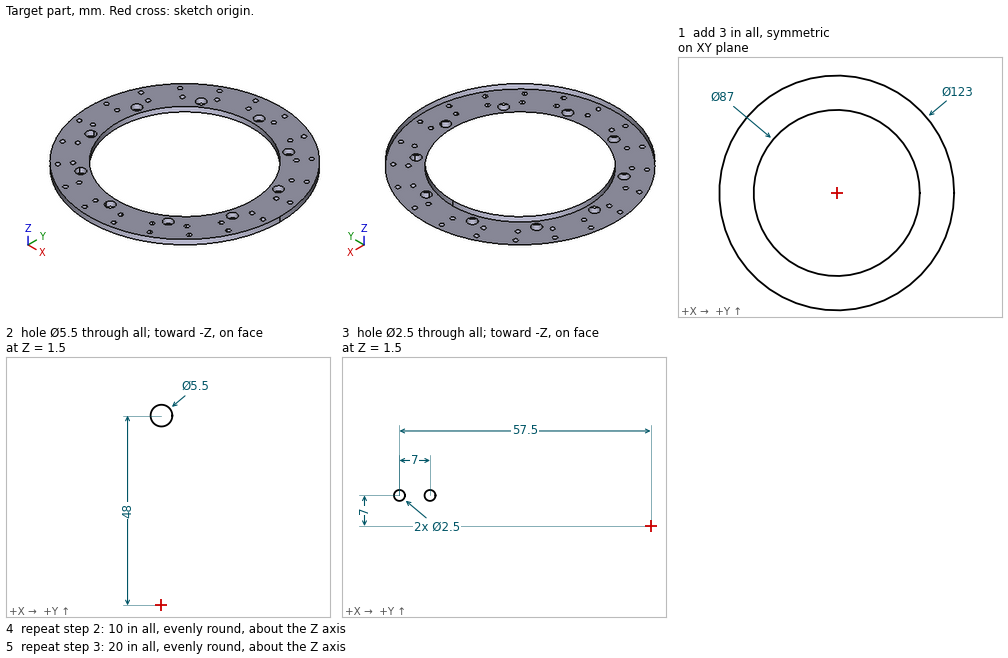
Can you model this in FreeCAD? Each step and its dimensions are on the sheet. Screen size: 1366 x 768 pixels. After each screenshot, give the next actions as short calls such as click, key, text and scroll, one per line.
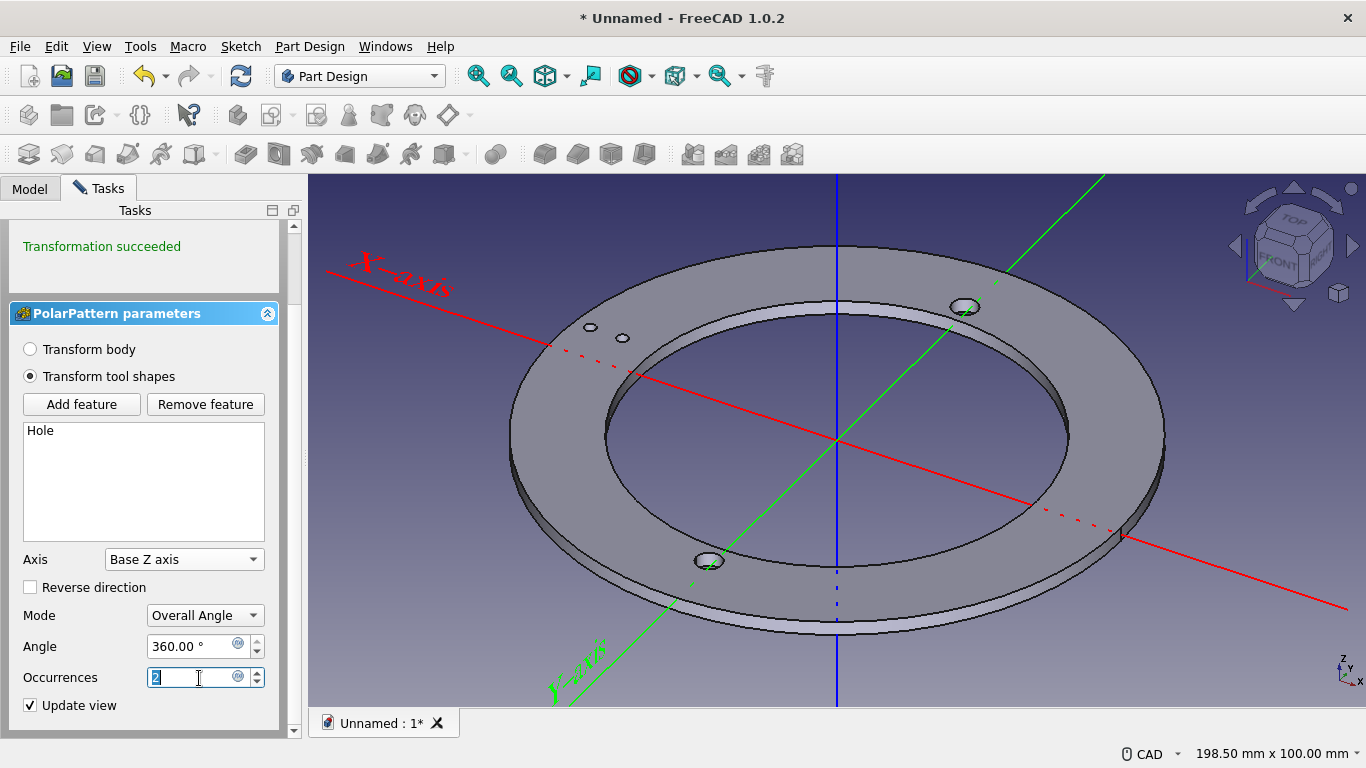
text(10)
key(Tab)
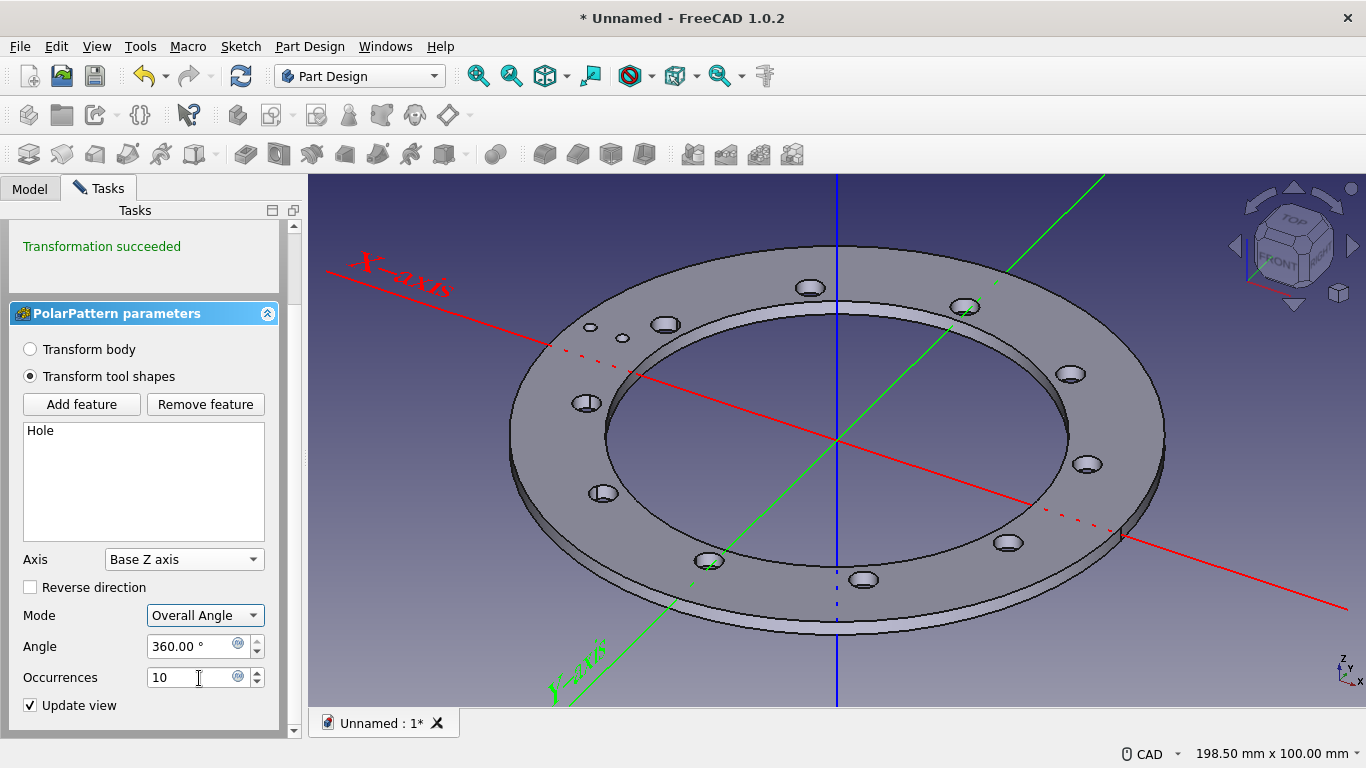
scroll(294, 479, up, 3)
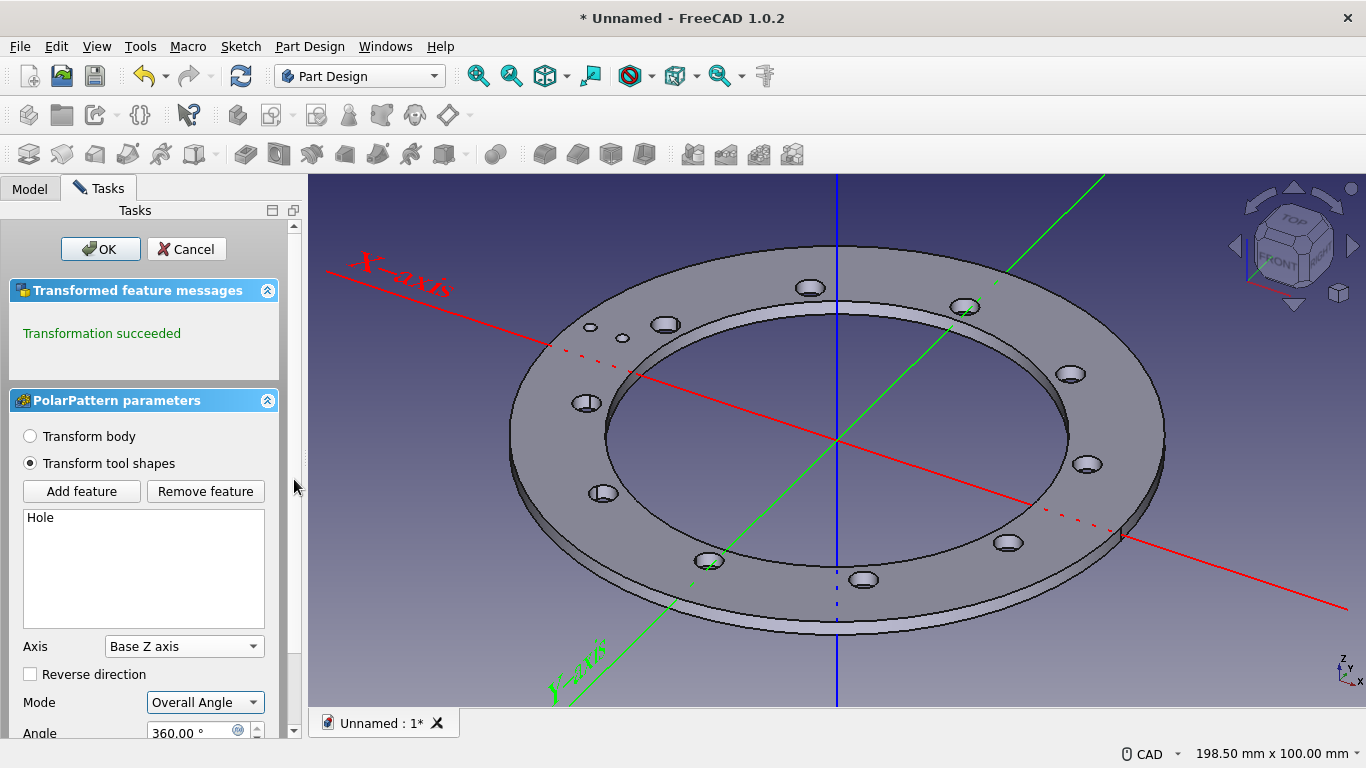
click(101, 249)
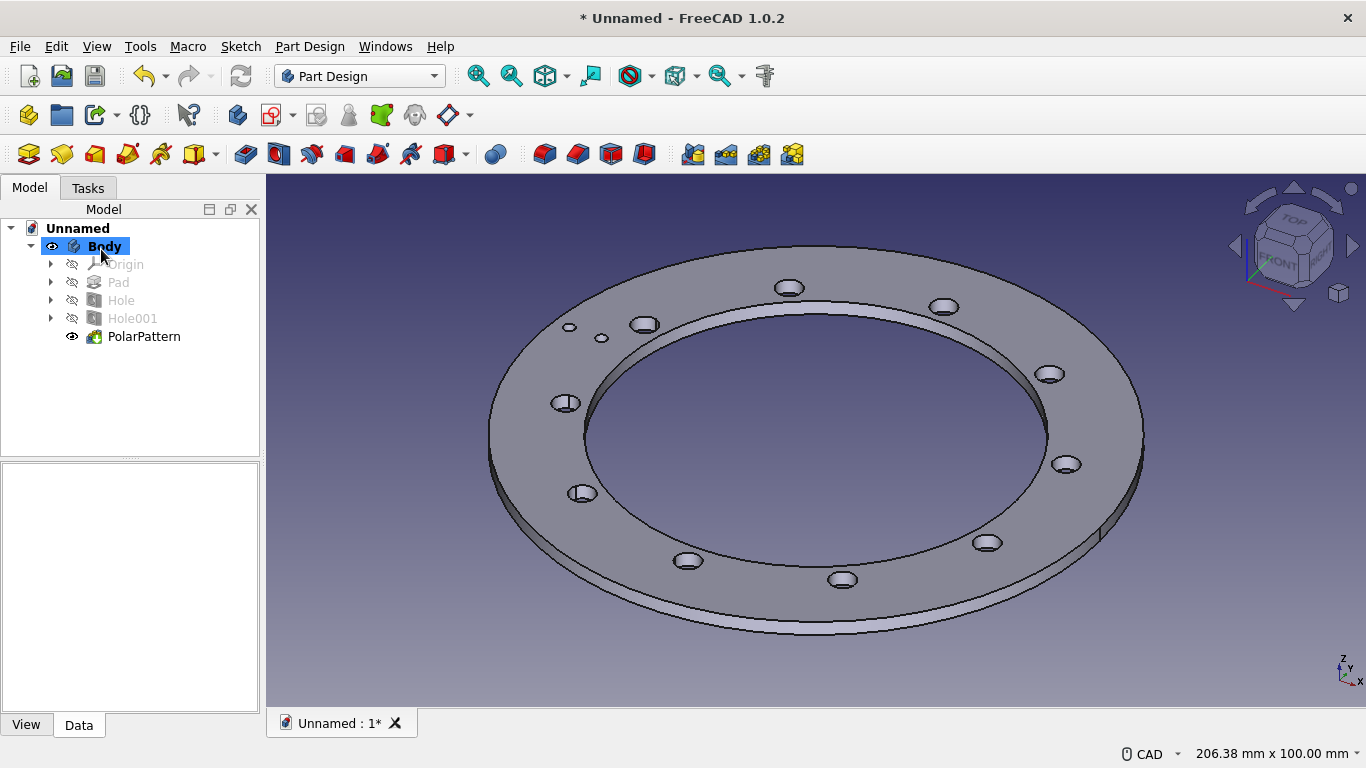
click(117, 318)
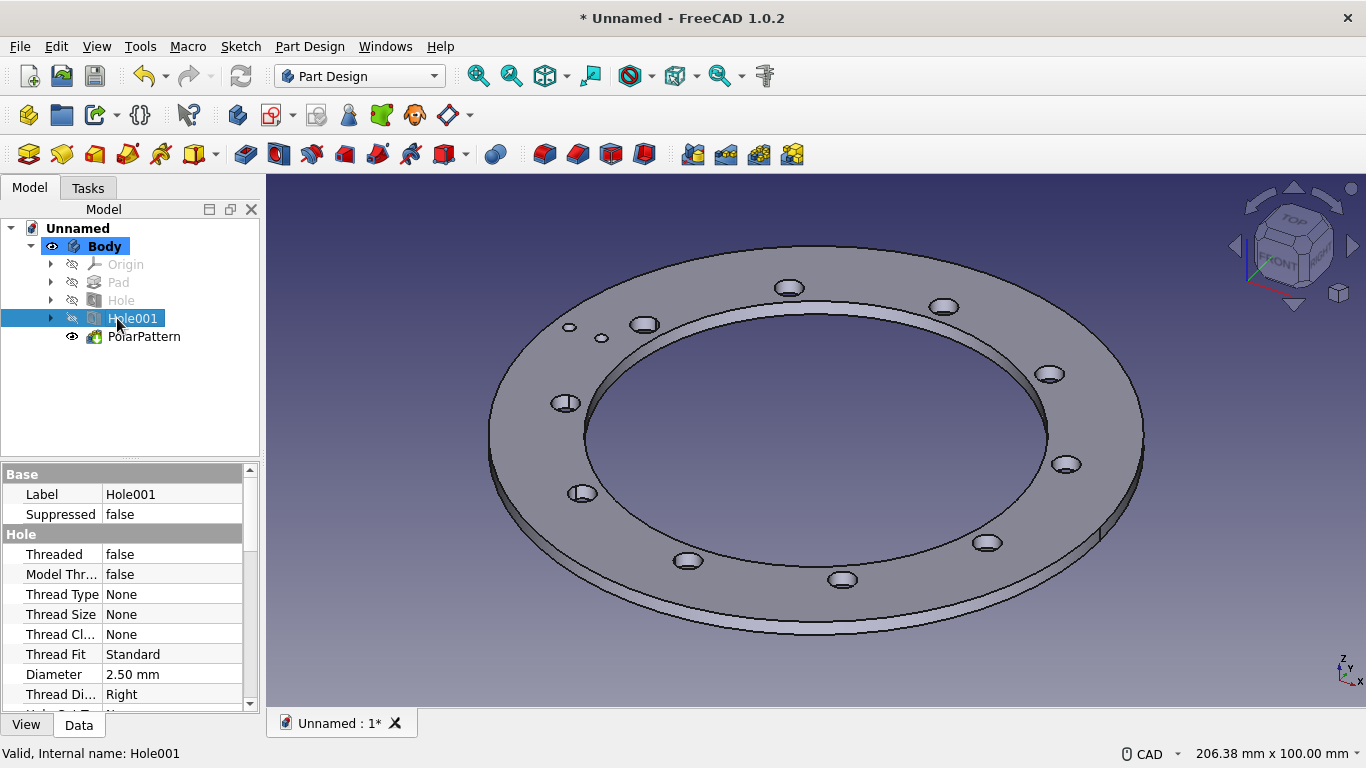
click(759, 154)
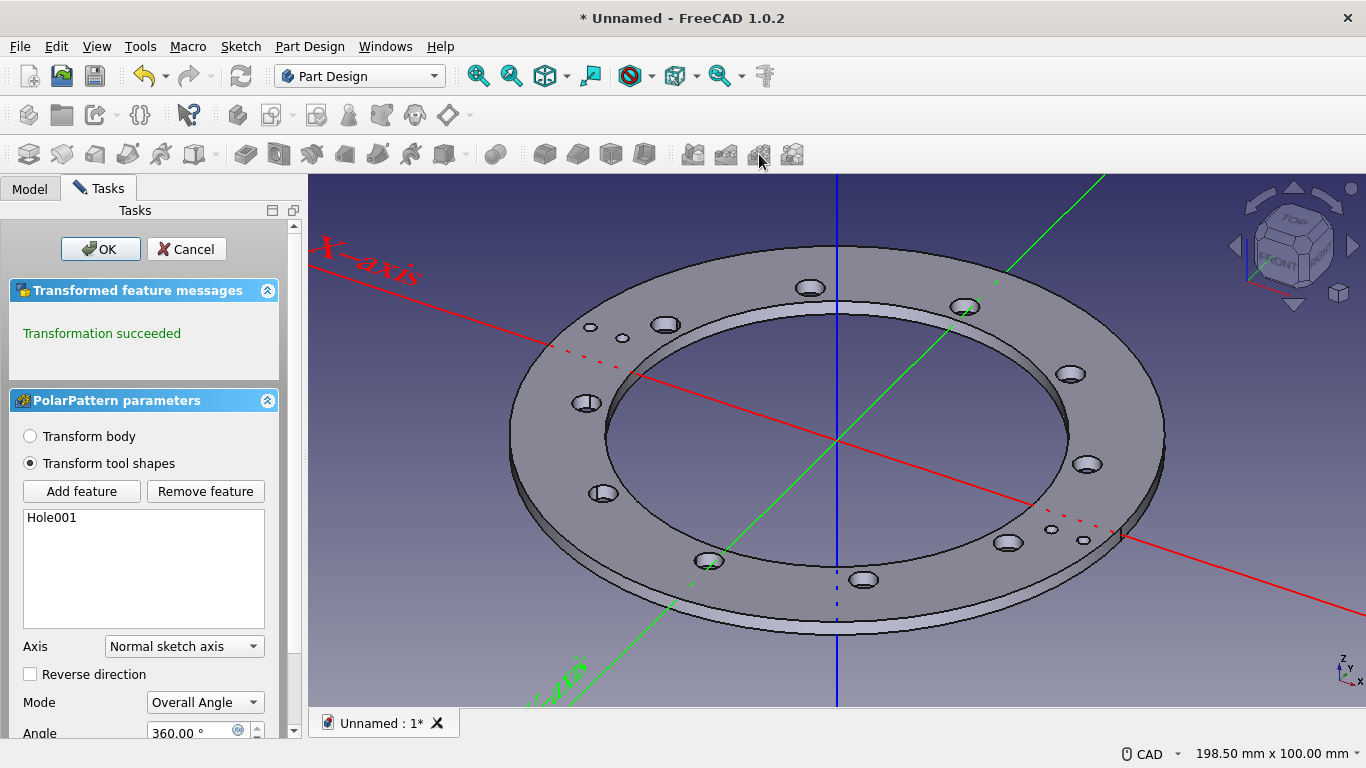
click(185, 646)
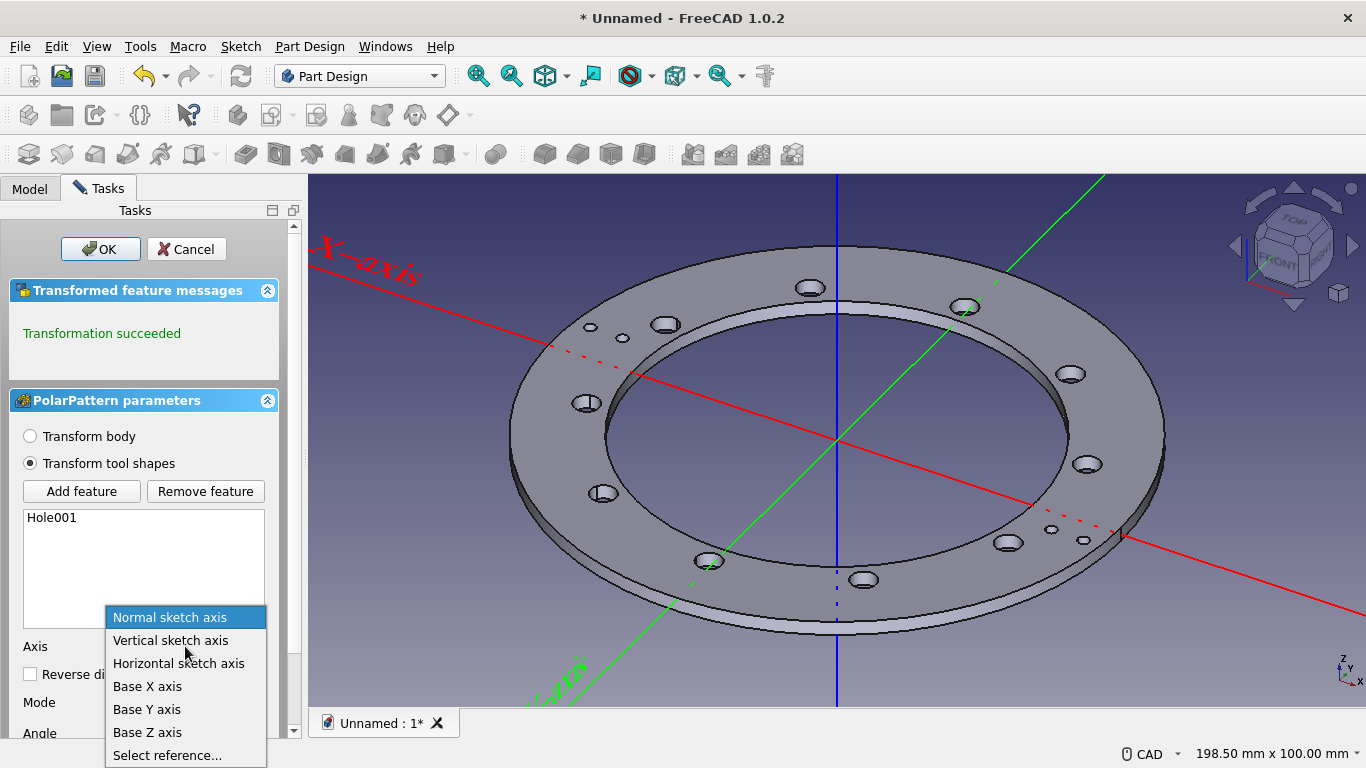
click(184, 732)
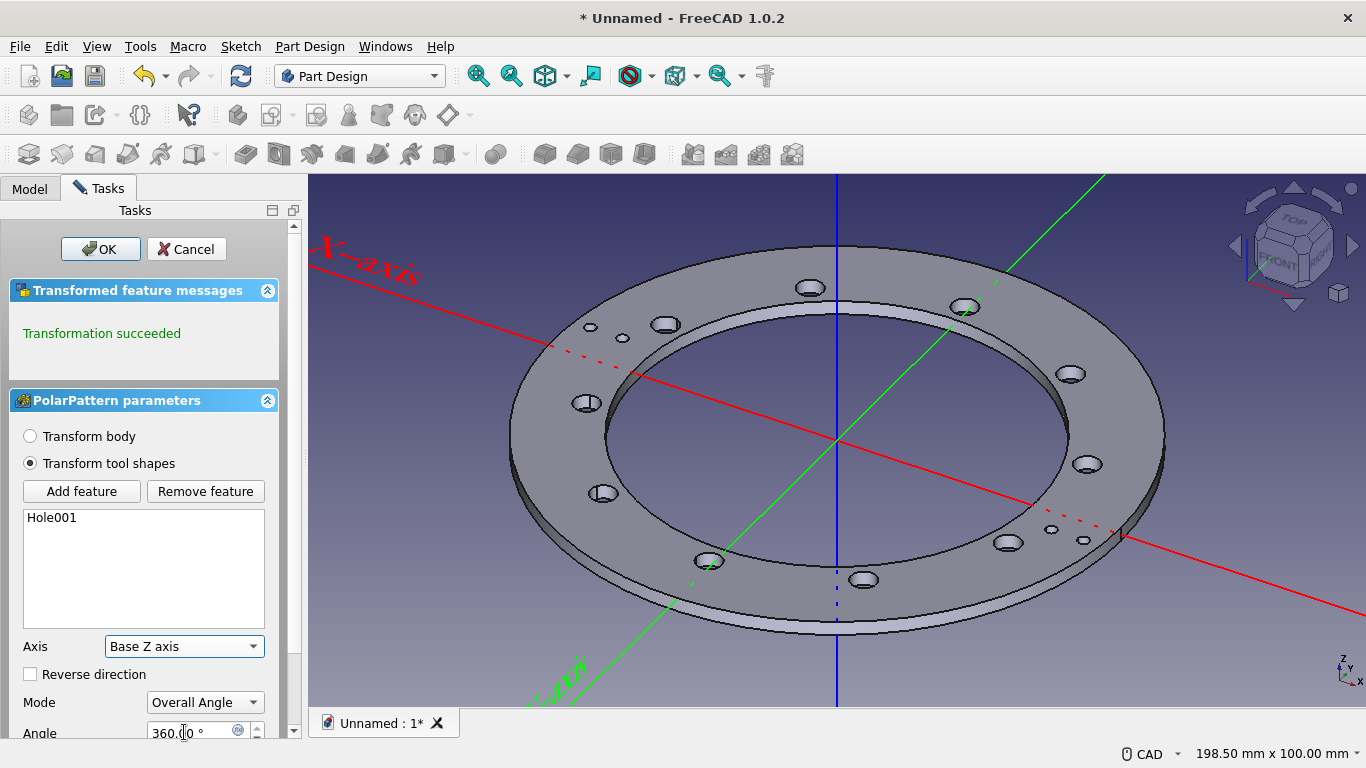
scroll(294, 479, down, 2)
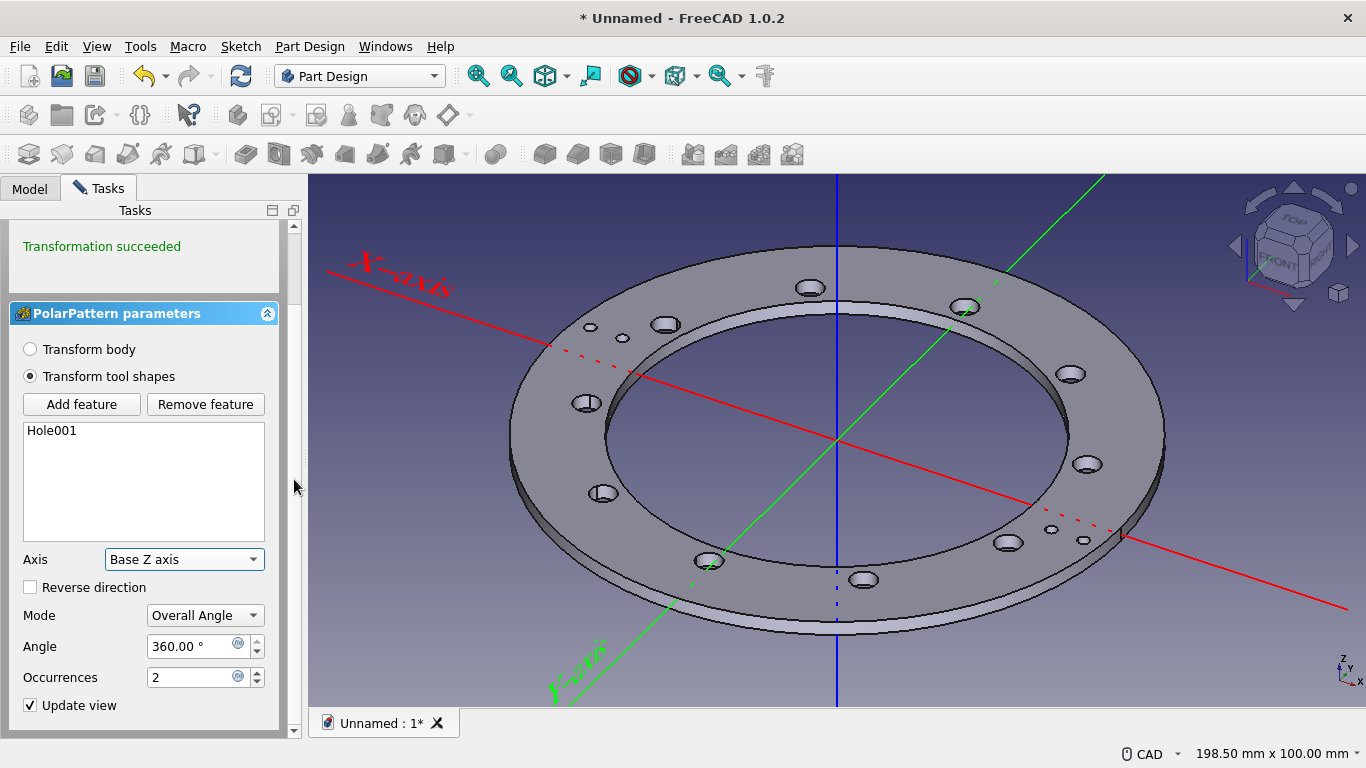
triple_click(199, 678)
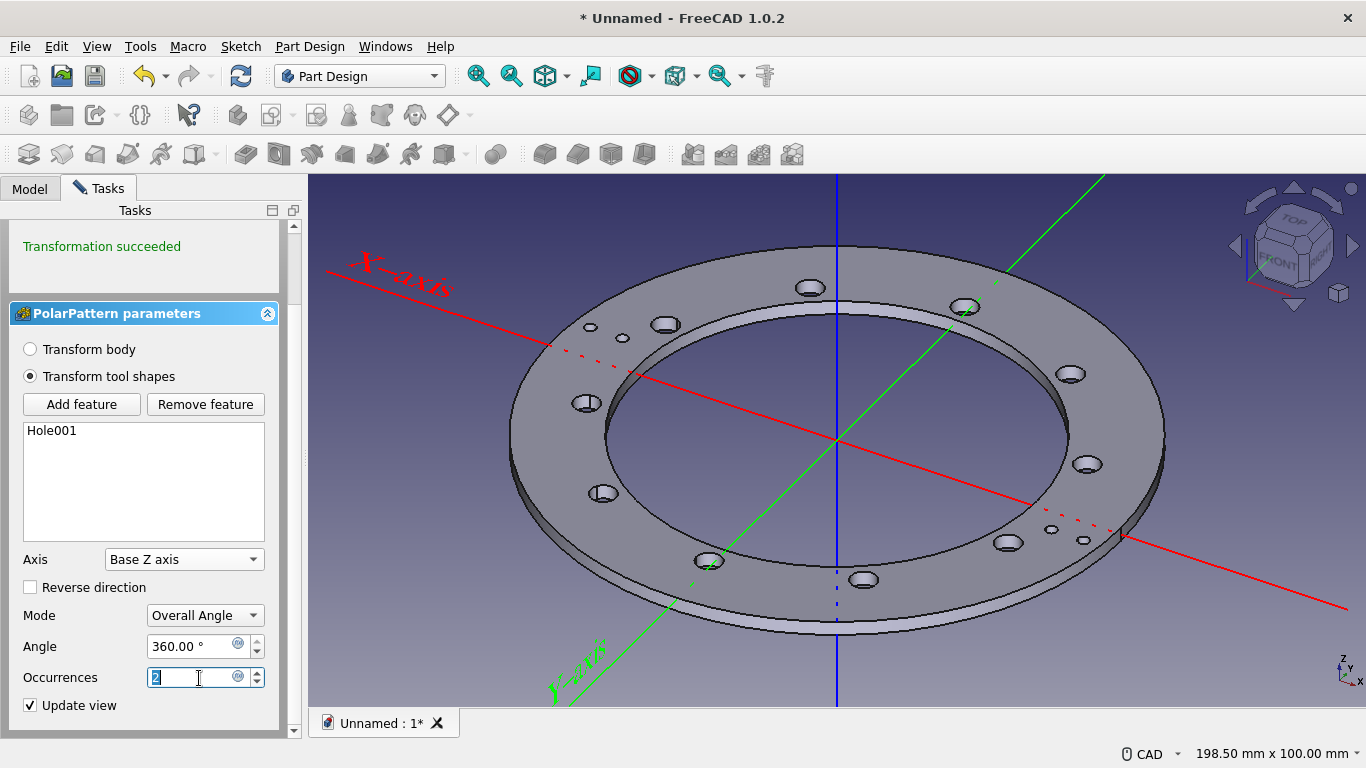
text(20)
key(Tab)